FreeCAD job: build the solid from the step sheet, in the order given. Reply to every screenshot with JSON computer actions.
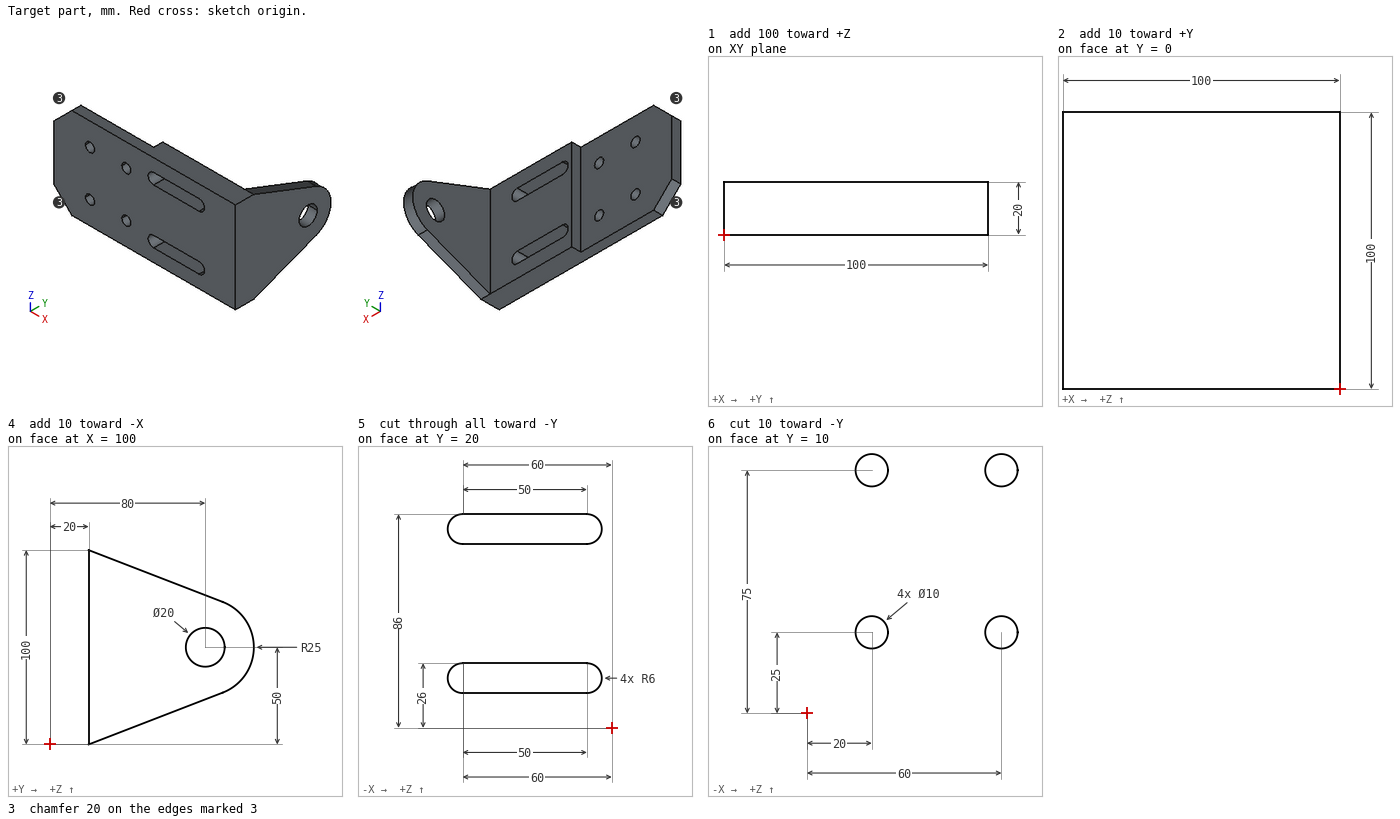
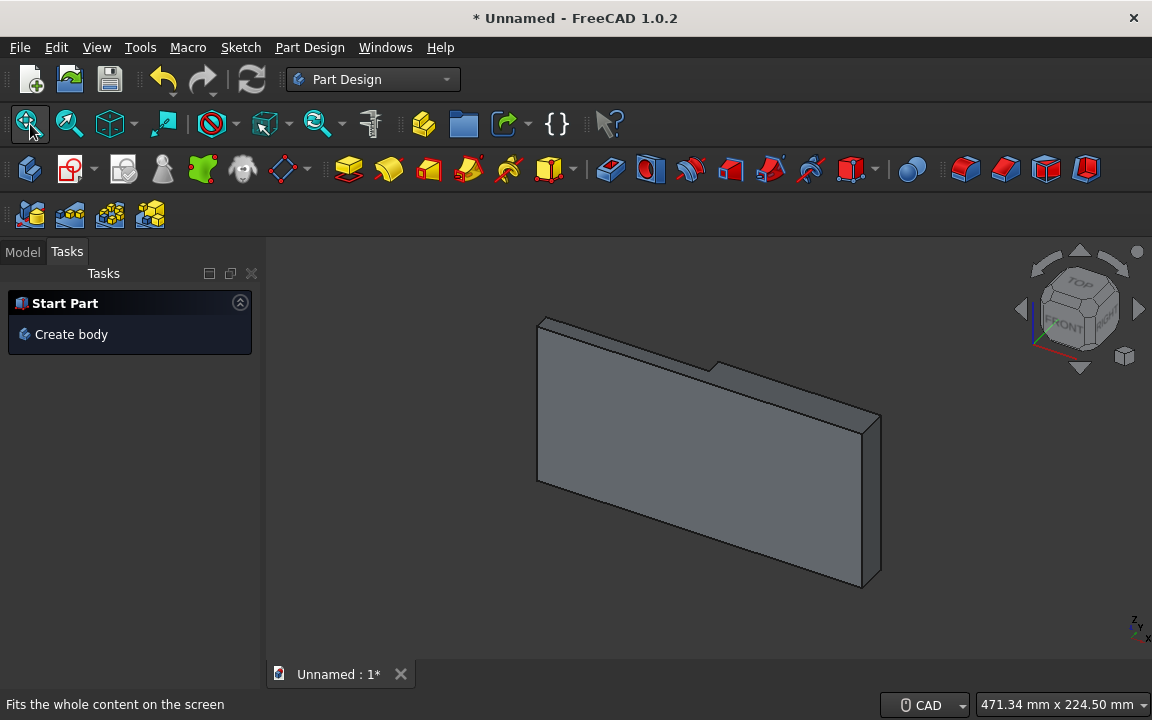
{"action": "key", "text": "0"}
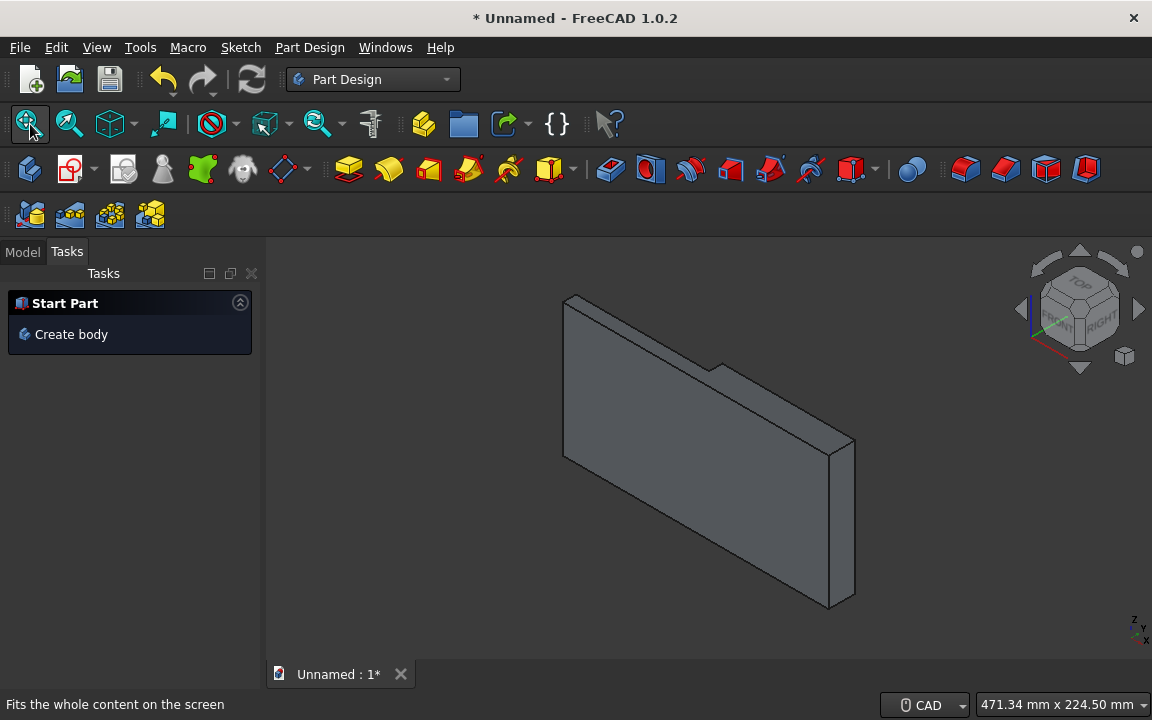
{"action": "scroll", "coordinate": [569, 451], "scroll_direction": "up", "scroll_amount": 4}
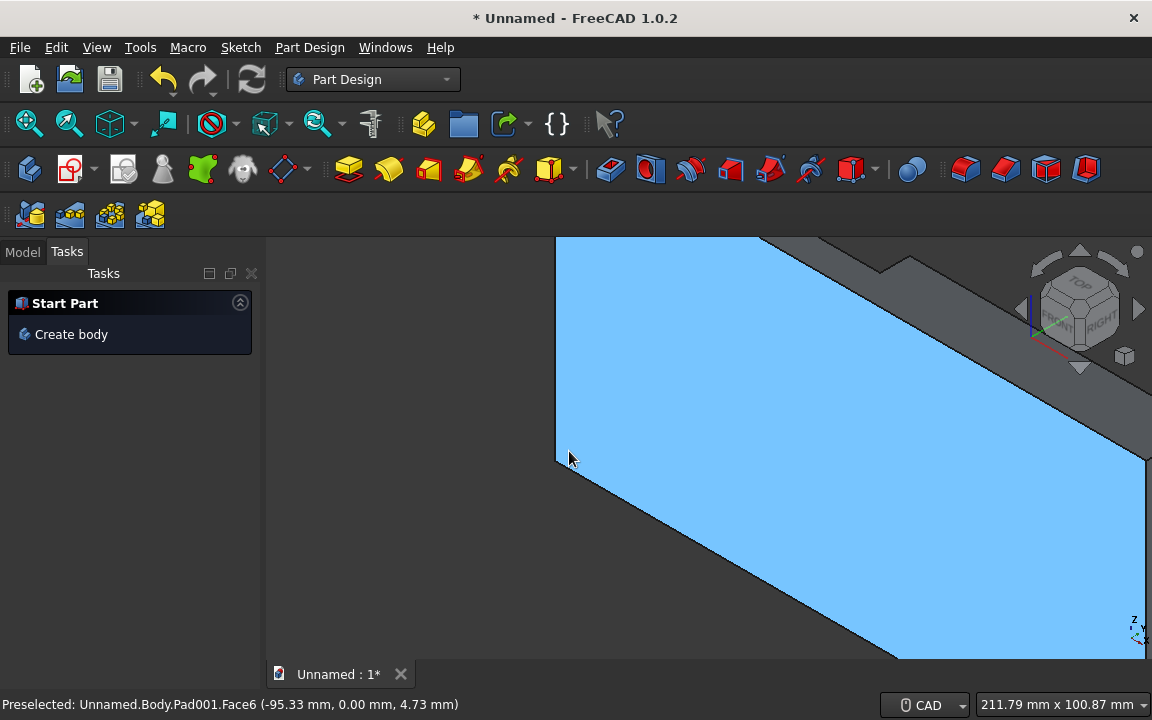
{"action": "left_click", "coordinate": [30, 124]}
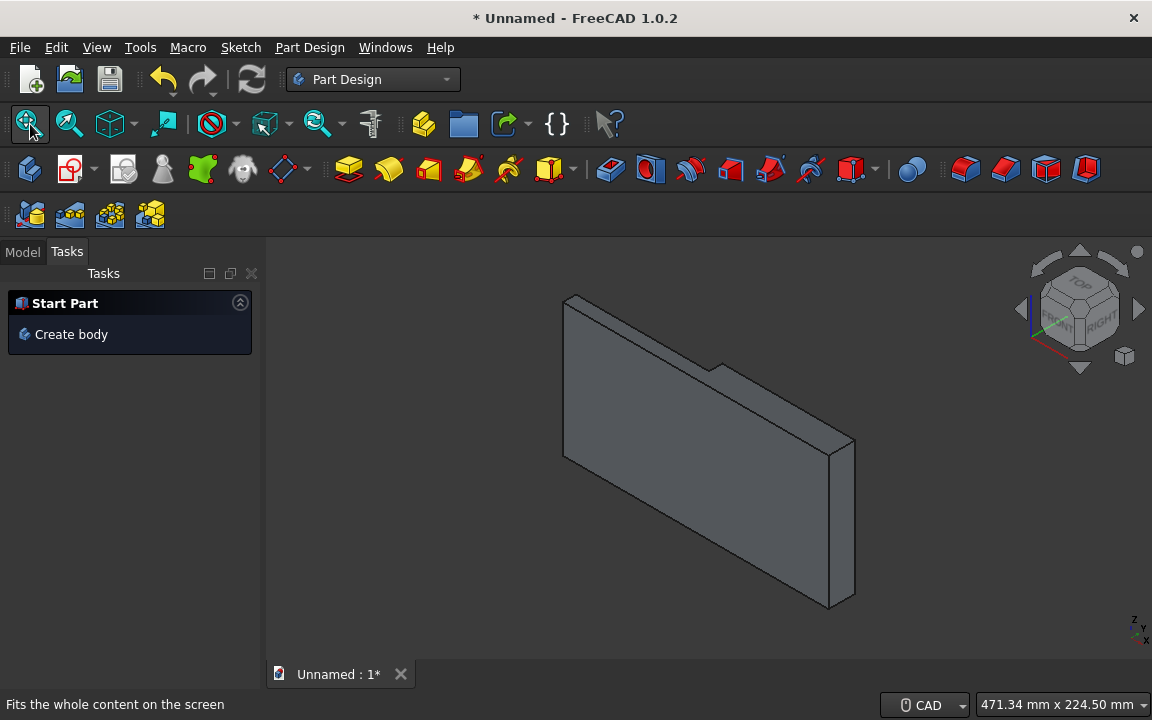
{"action": "key", "text": "2"}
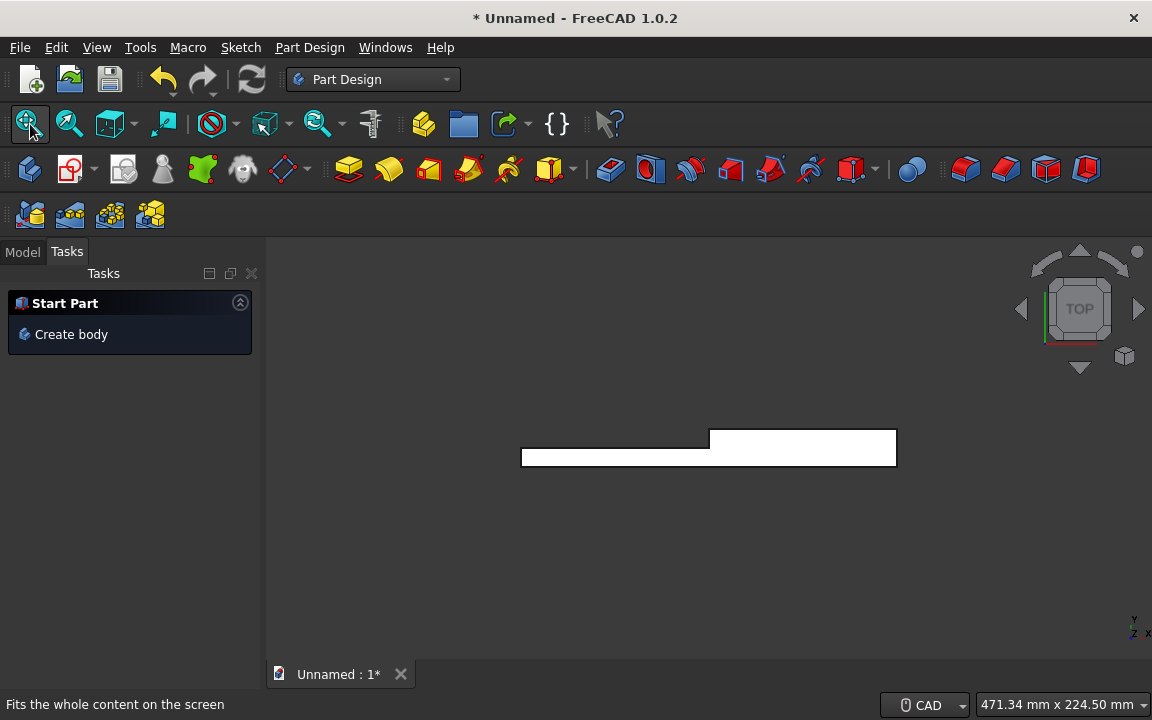
{"action": "left_click", "coordinate": [30, 124]}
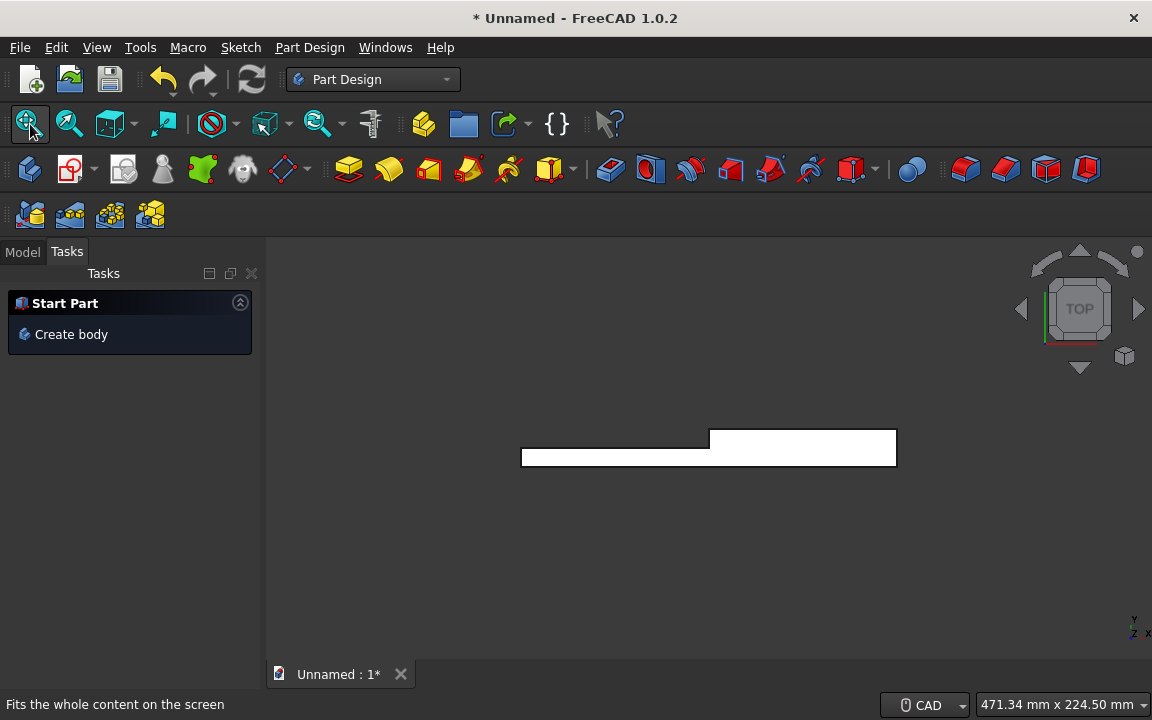
{"action": "left_click", "coordinate": [521, 456]}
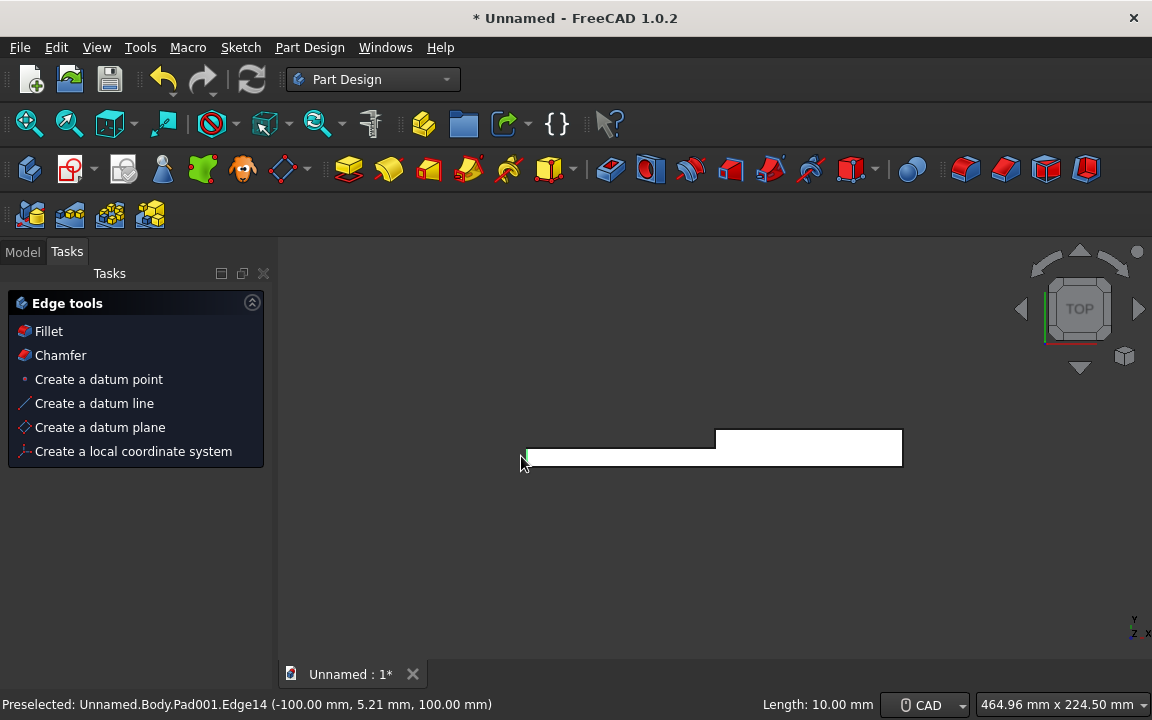
{"action": "scroll", "coordinate": [527, 456], "scroll_direction": "up", "scroll_amount": 4}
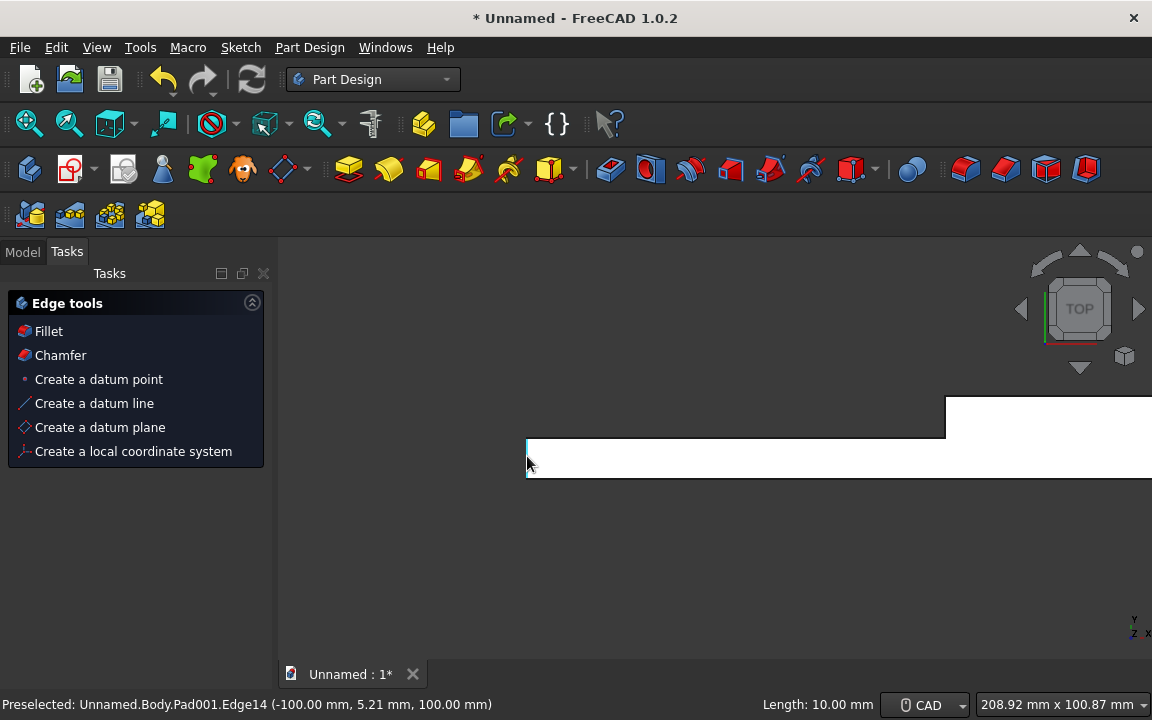
{"action": "left_click", "coordinate": [30, 124]}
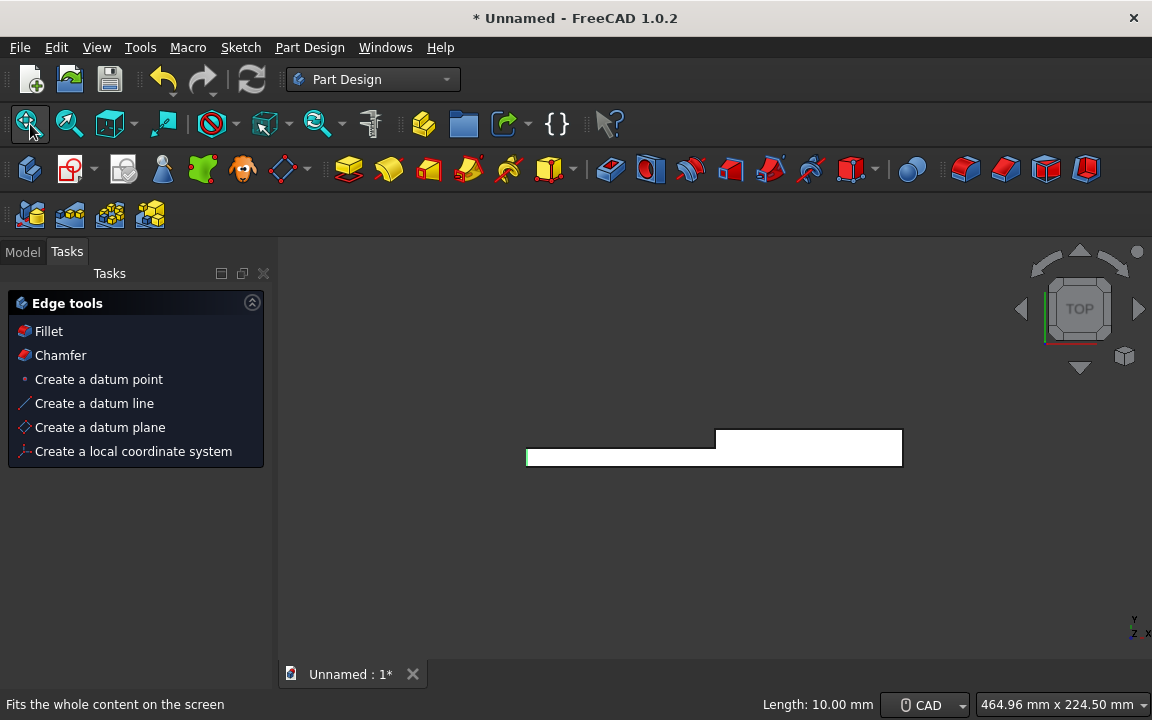
{"action": "key", "text": "1"}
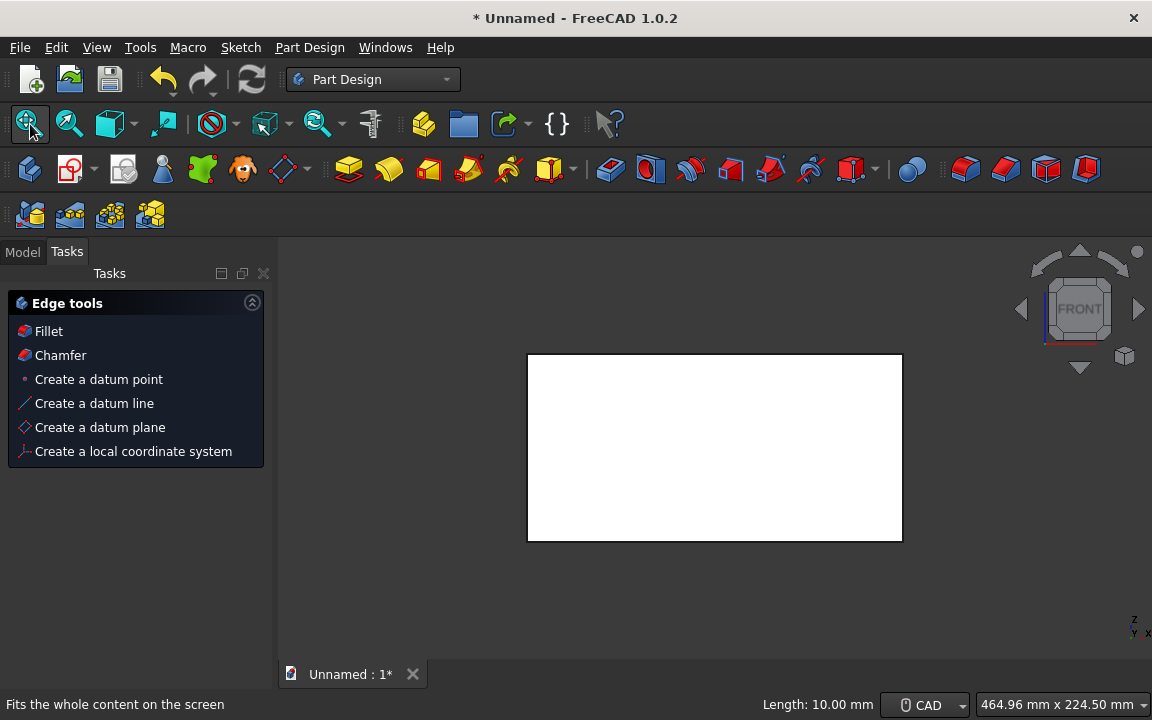
{"action": "left_click", "coordinate": [30, 124]}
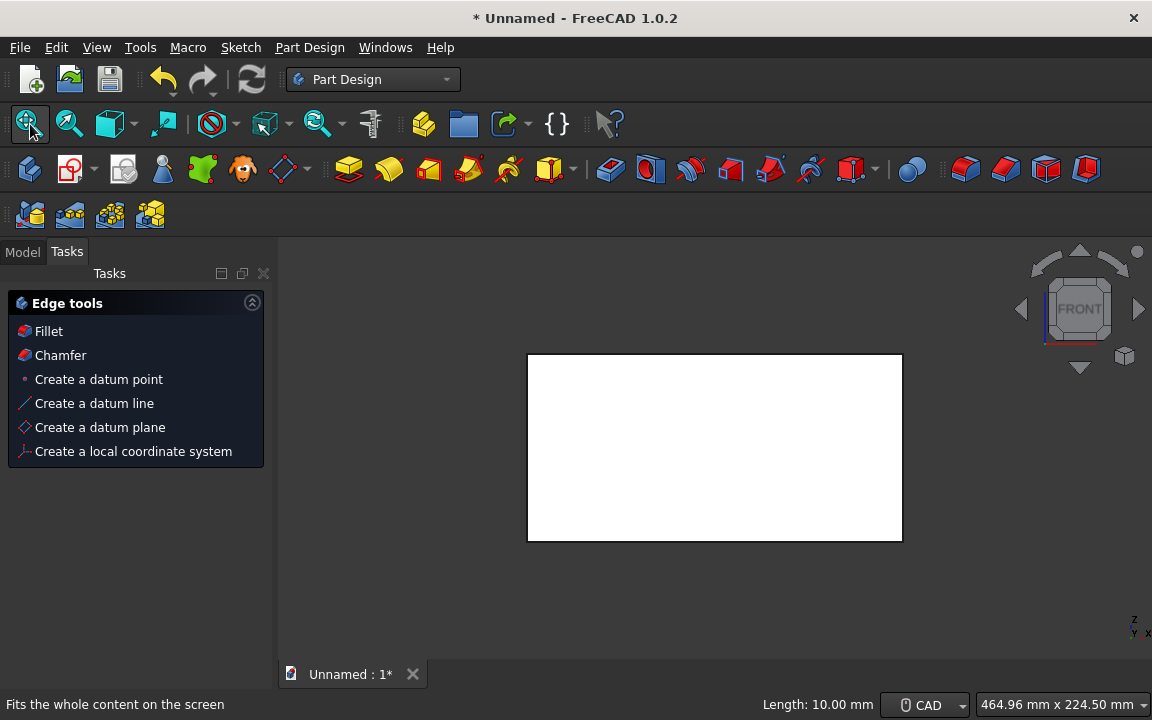
{"action": "scroll", "coordinate": [527, 541], "scroll_direction": "up", "scroll_amount": 4}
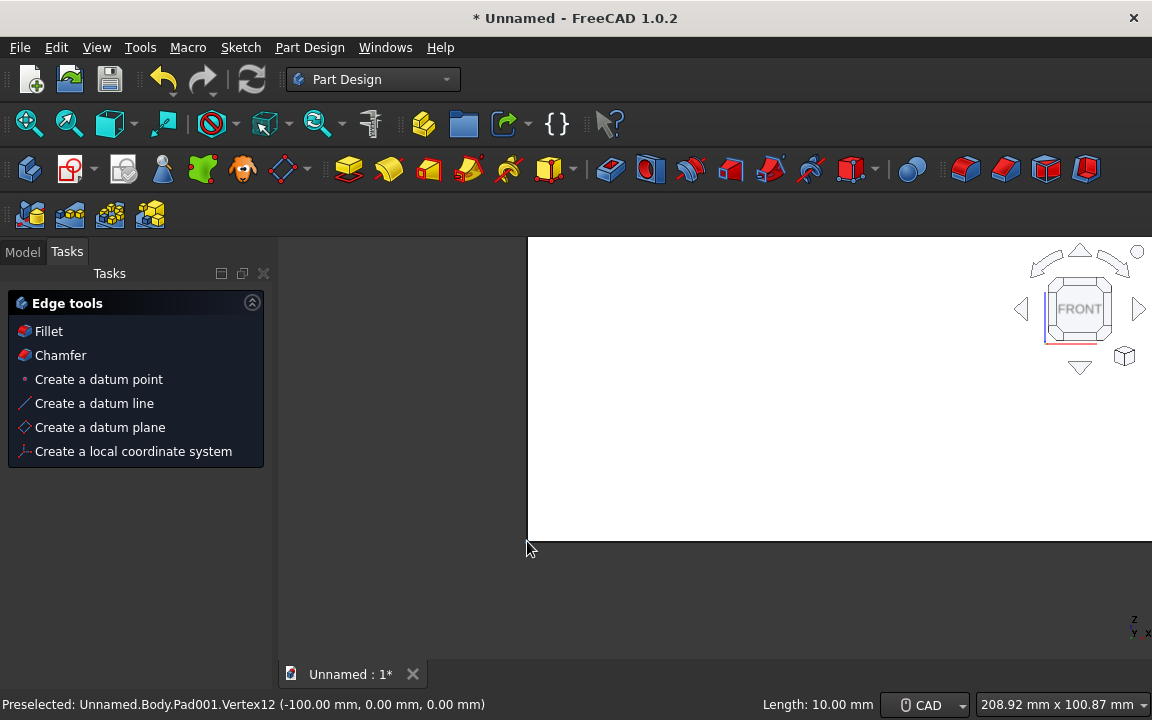
{"action": "left_click", "coordinate": [30, 124]}